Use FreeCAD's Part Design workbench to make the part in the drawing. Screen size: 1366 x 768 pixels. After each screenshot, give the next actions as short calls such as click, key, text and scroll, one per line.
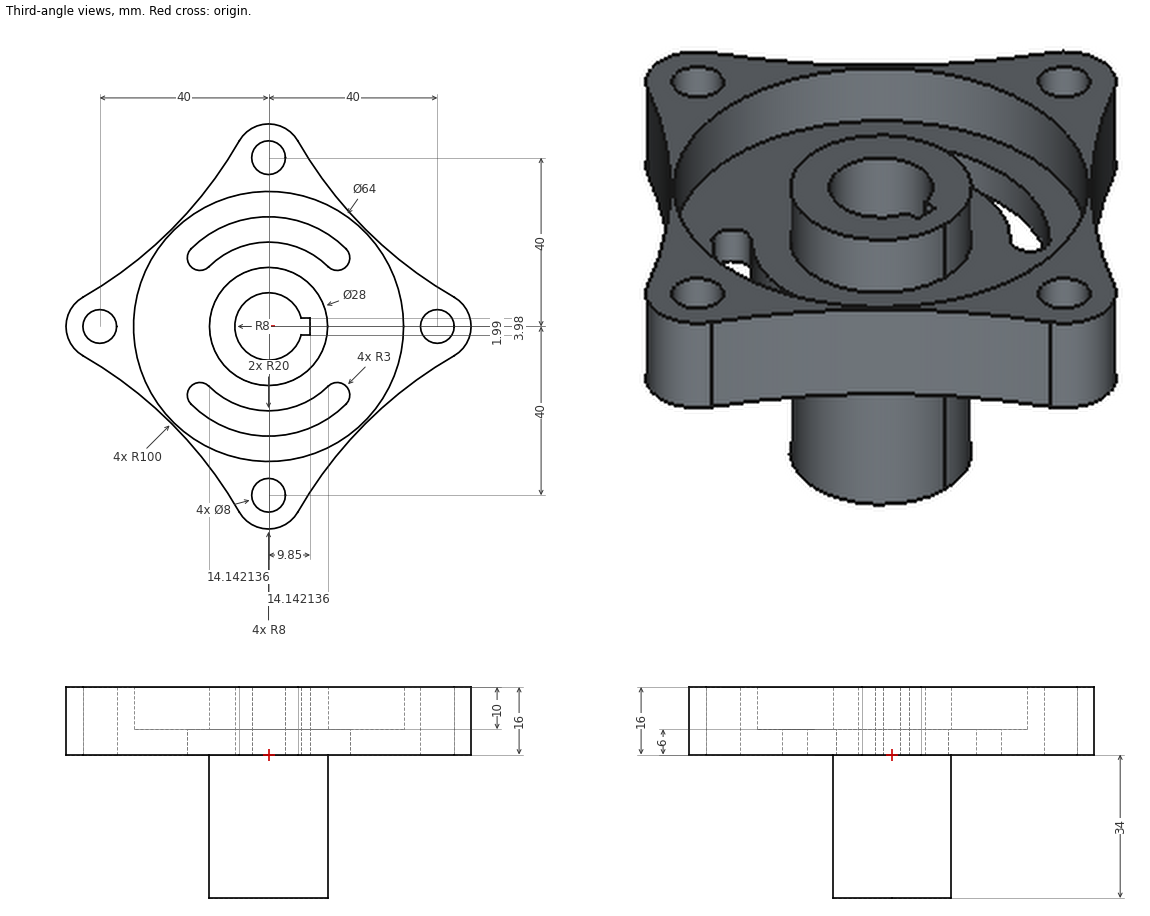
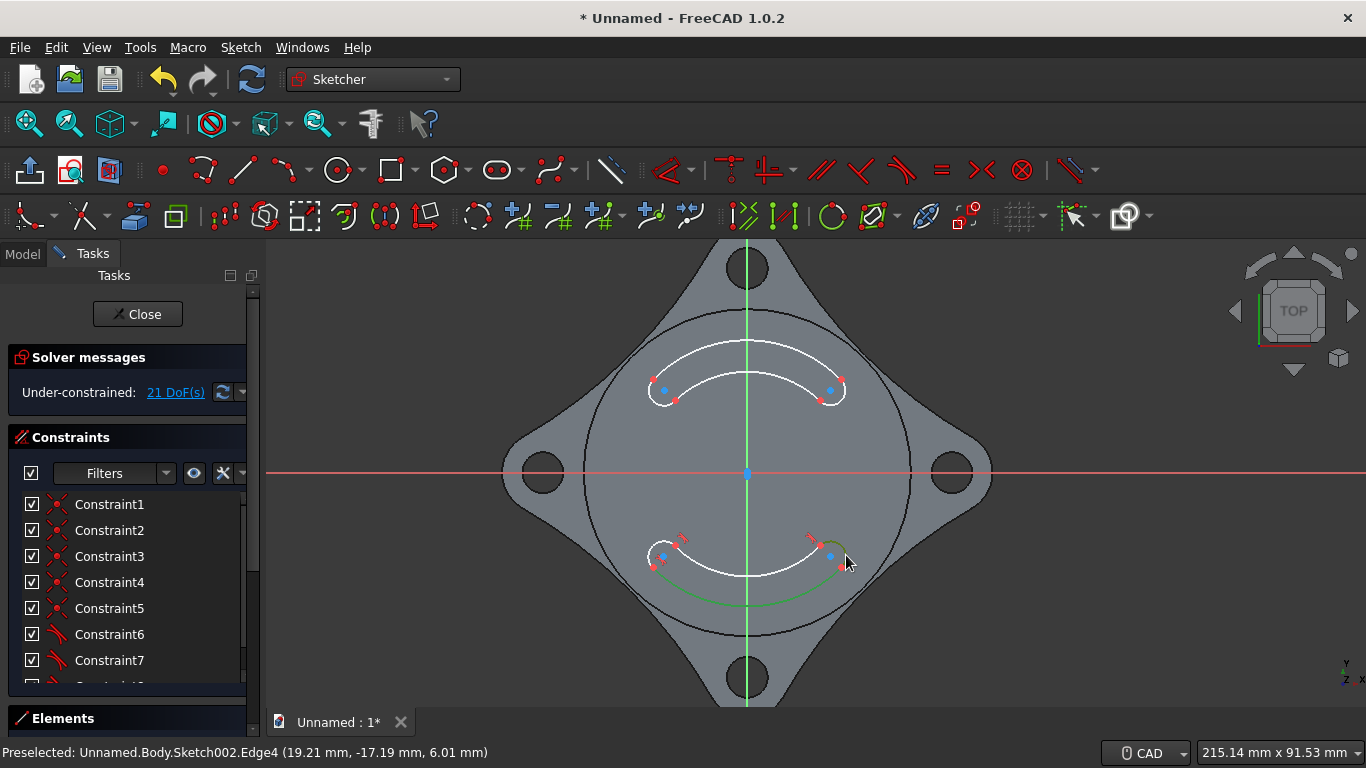
click(902, 170)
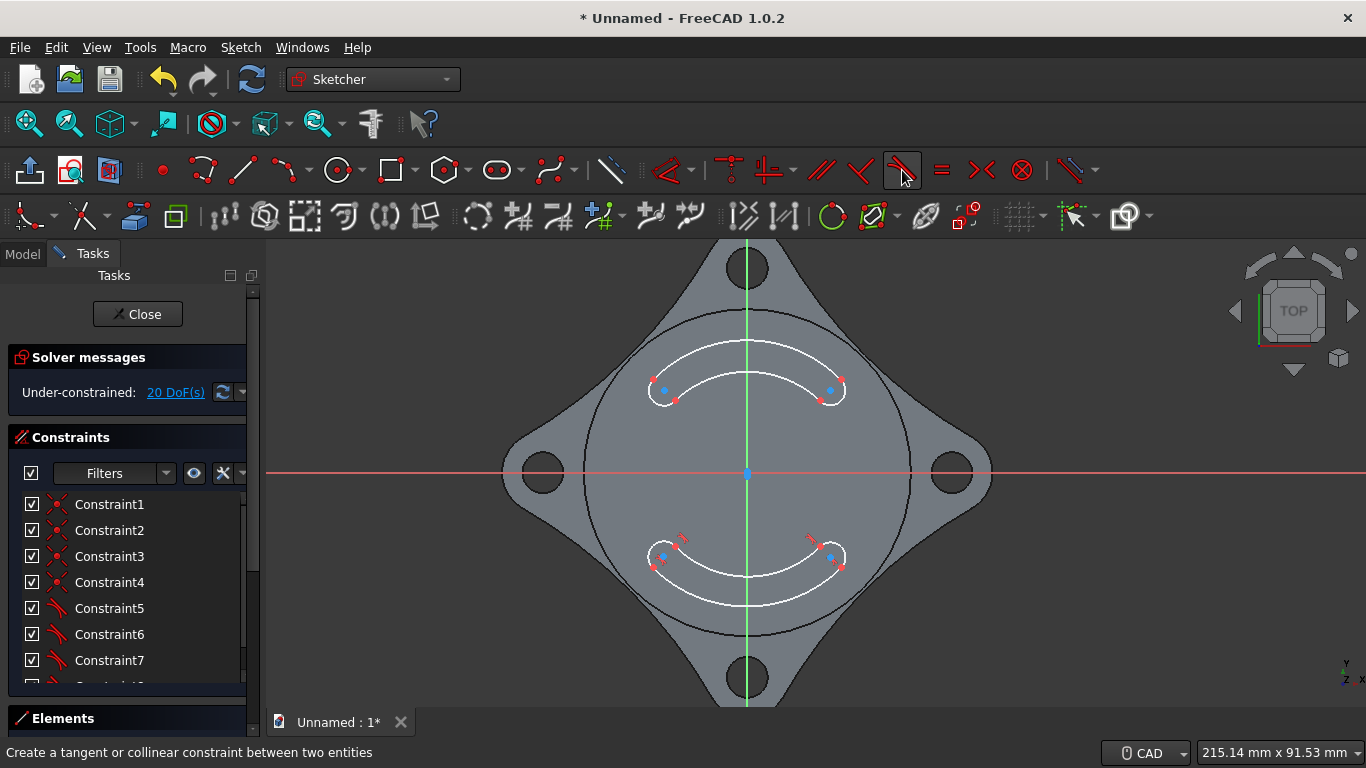
click(779, 377)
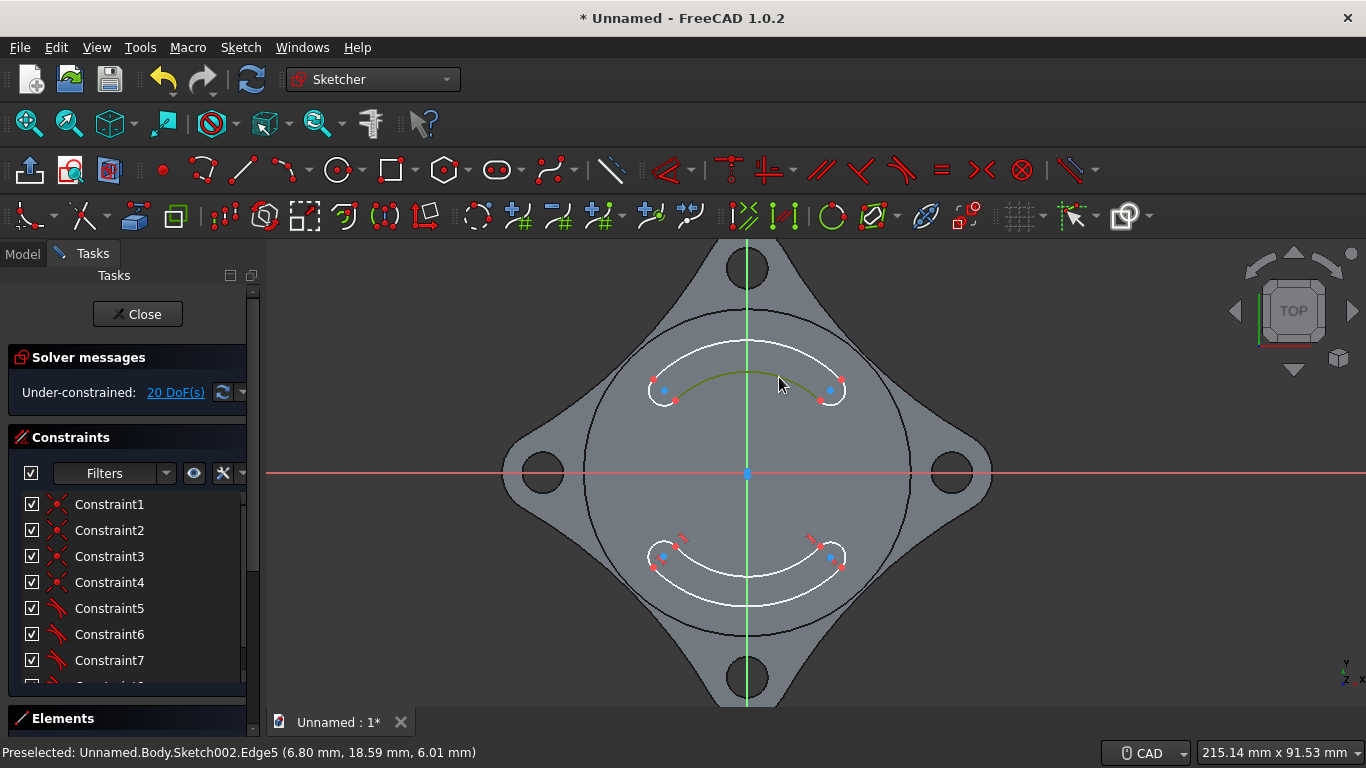
click(833, 405)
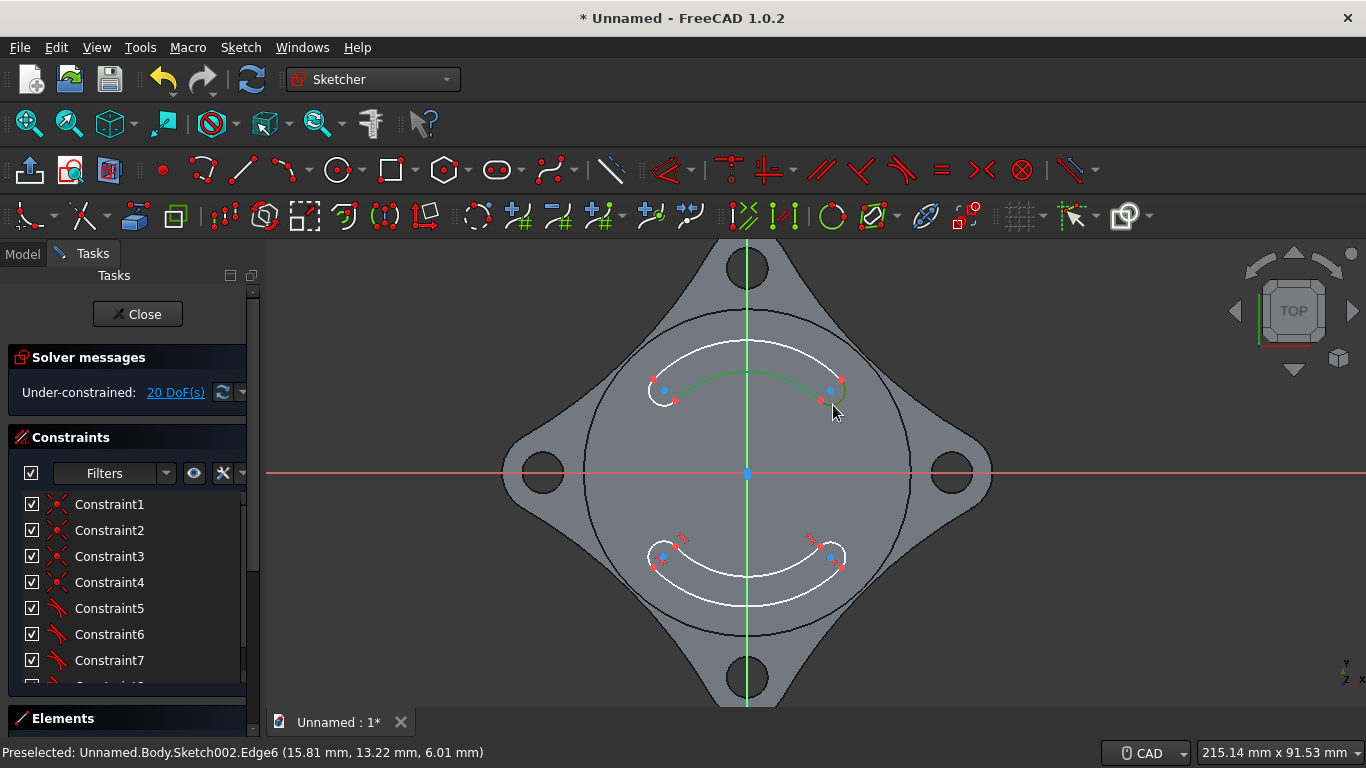
key(t)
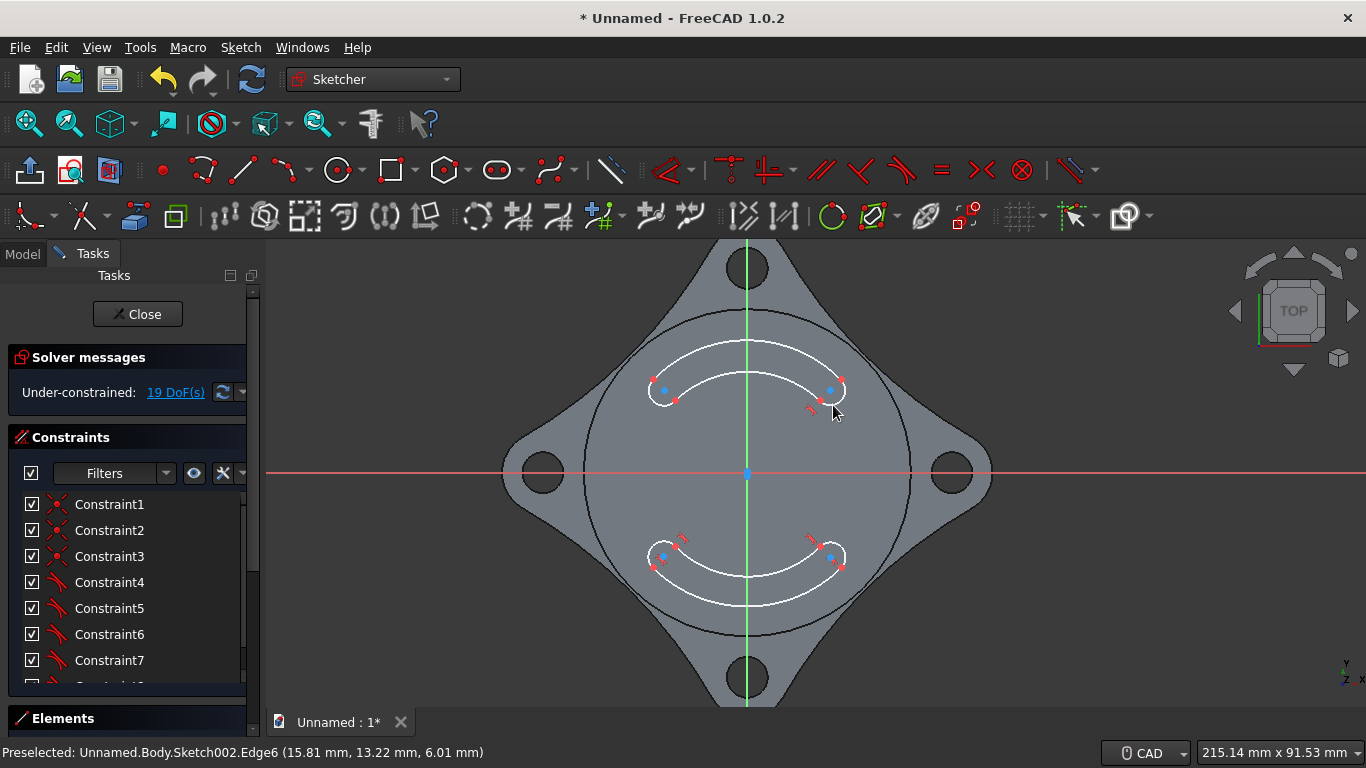
click(779, 377)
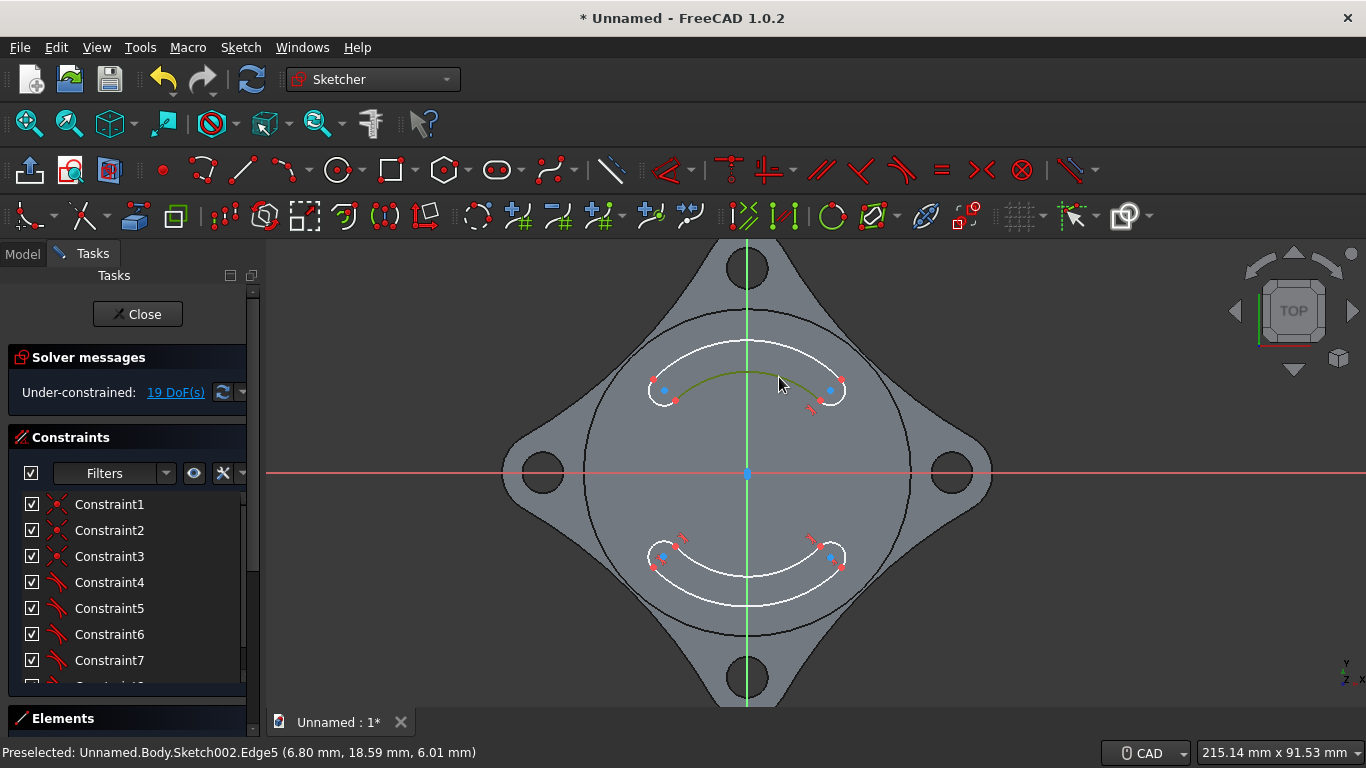
click(649, 393)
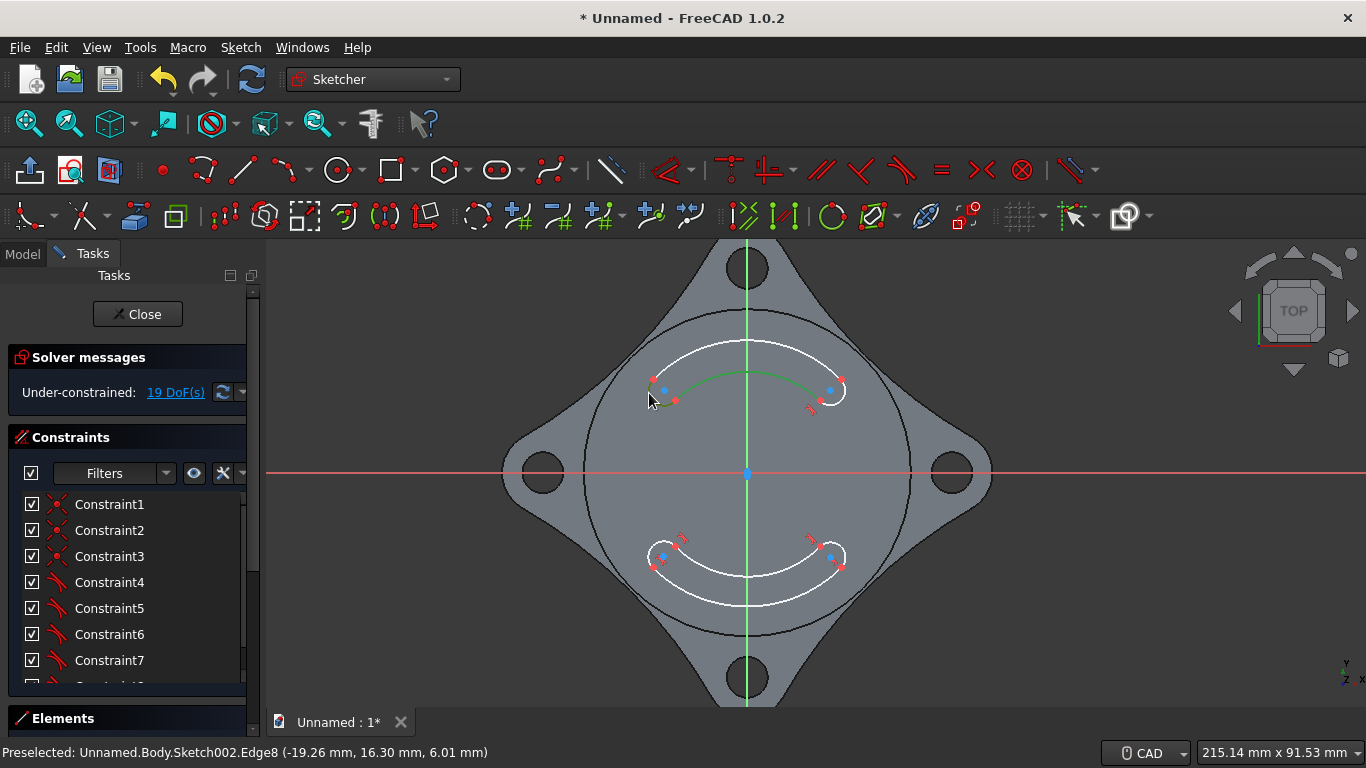
click(902, 170)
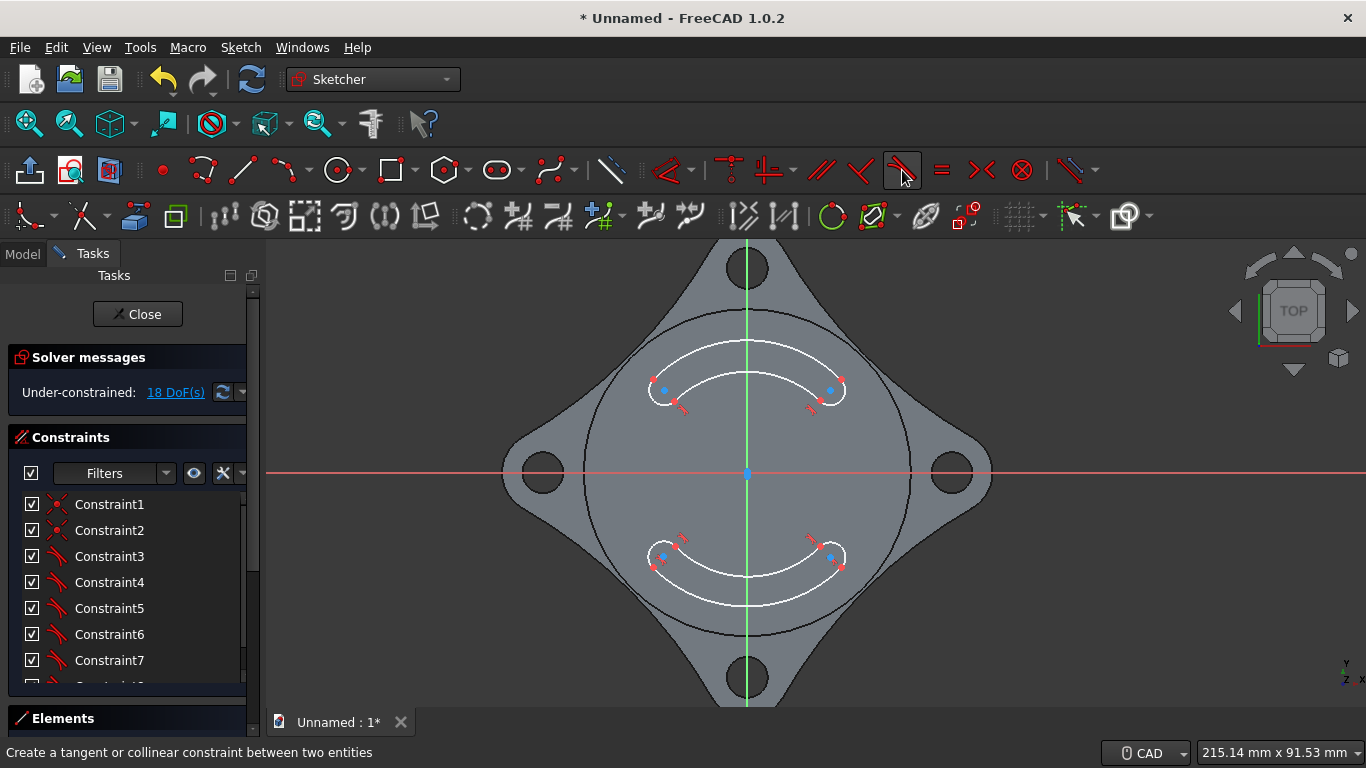
click(833, 405)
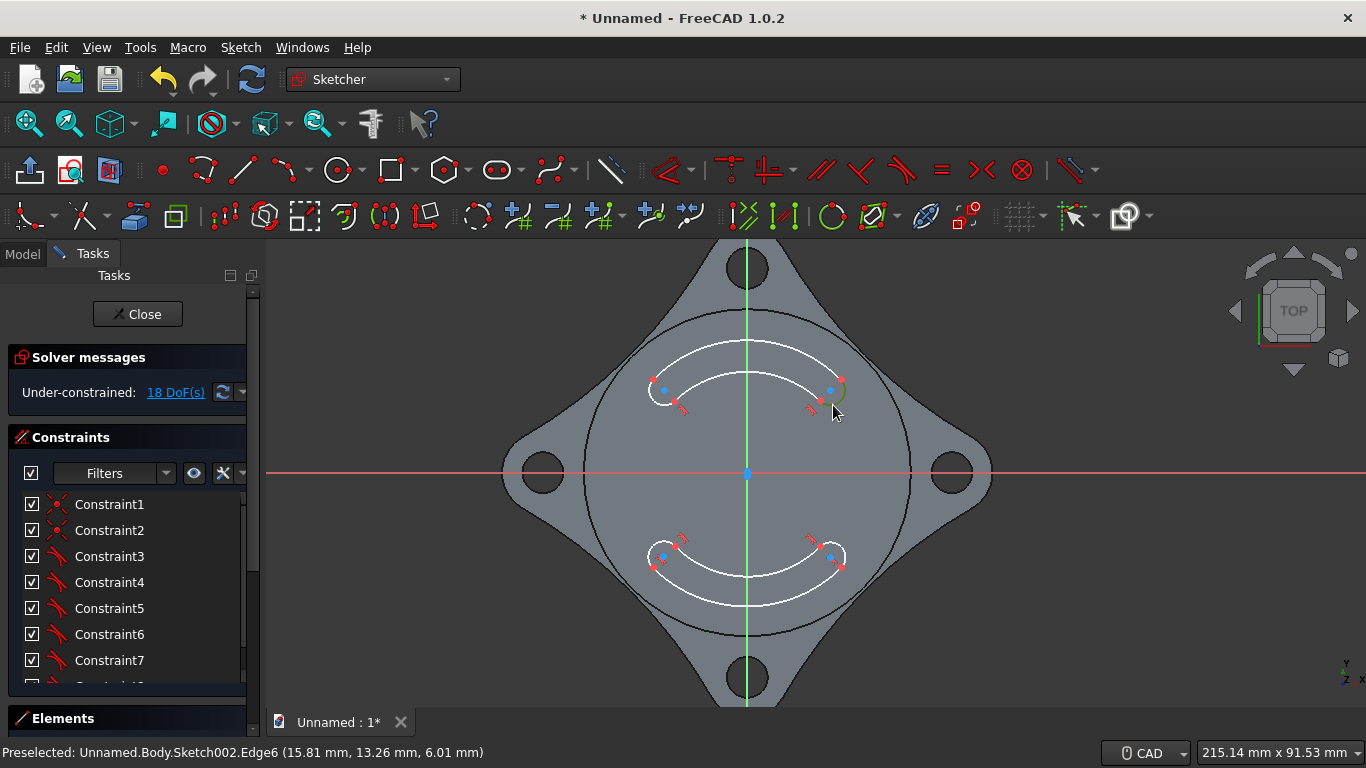
click(788, 347)